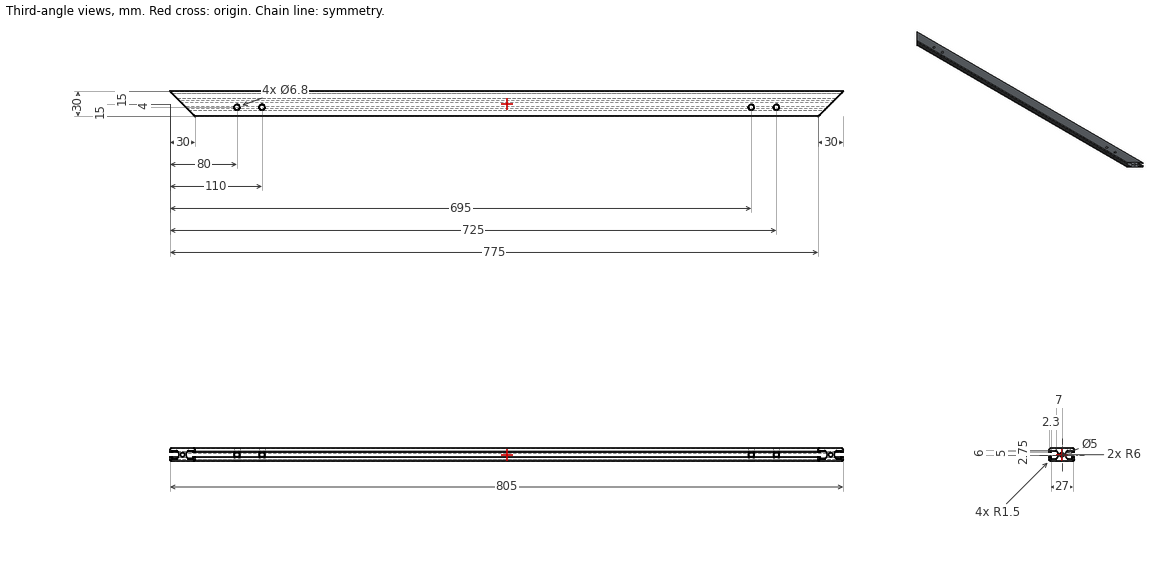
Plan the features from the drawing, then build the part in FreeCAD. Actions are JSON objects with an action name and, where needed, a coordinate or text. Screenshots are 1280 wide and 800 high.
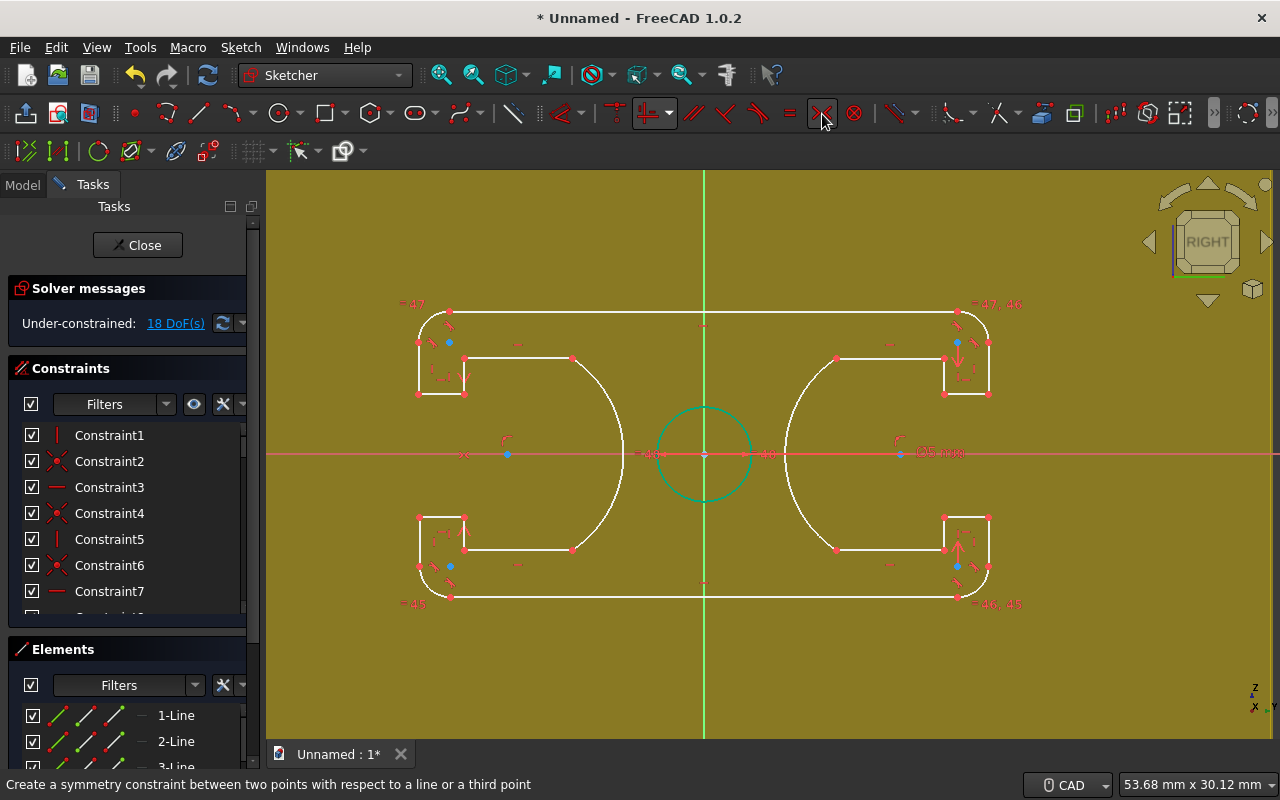
{"action": "left_click", "coordinate": [419, 394]}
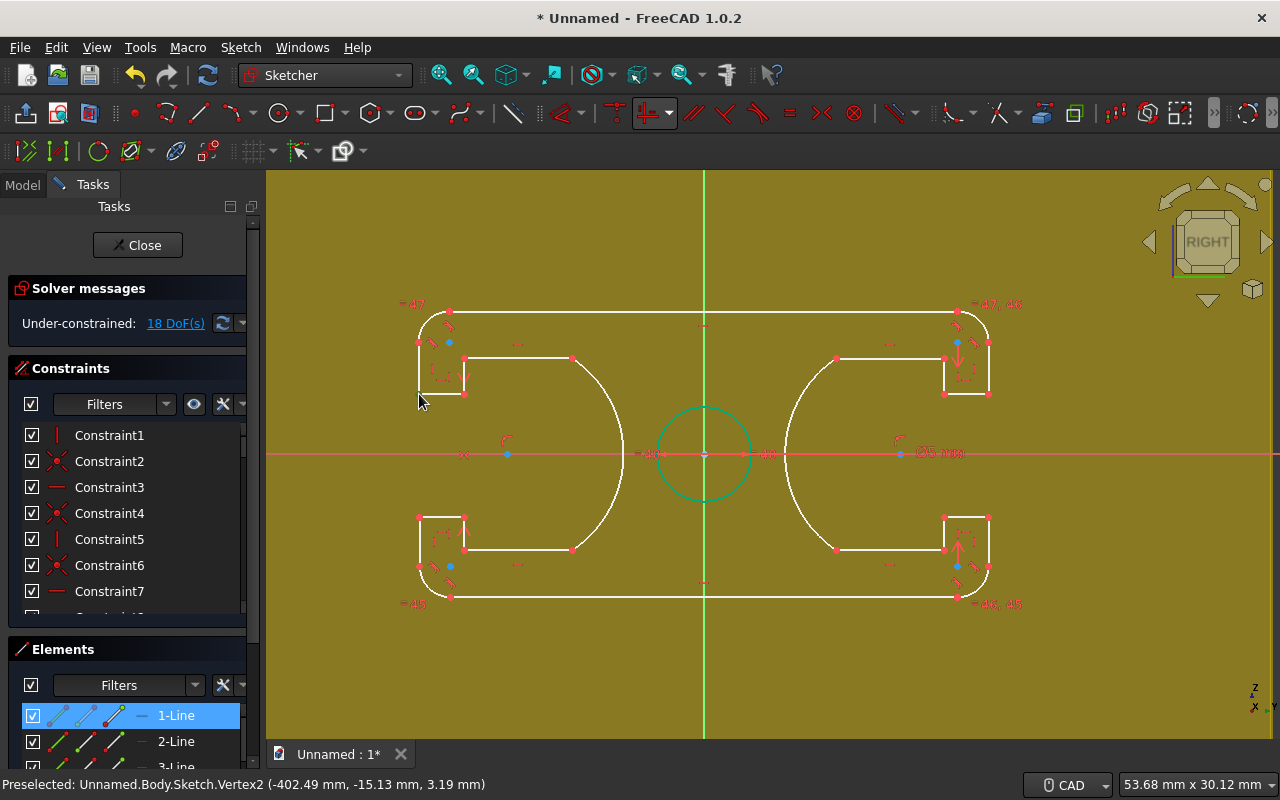
{"action": "left_click", "coordinate": [420, 517]}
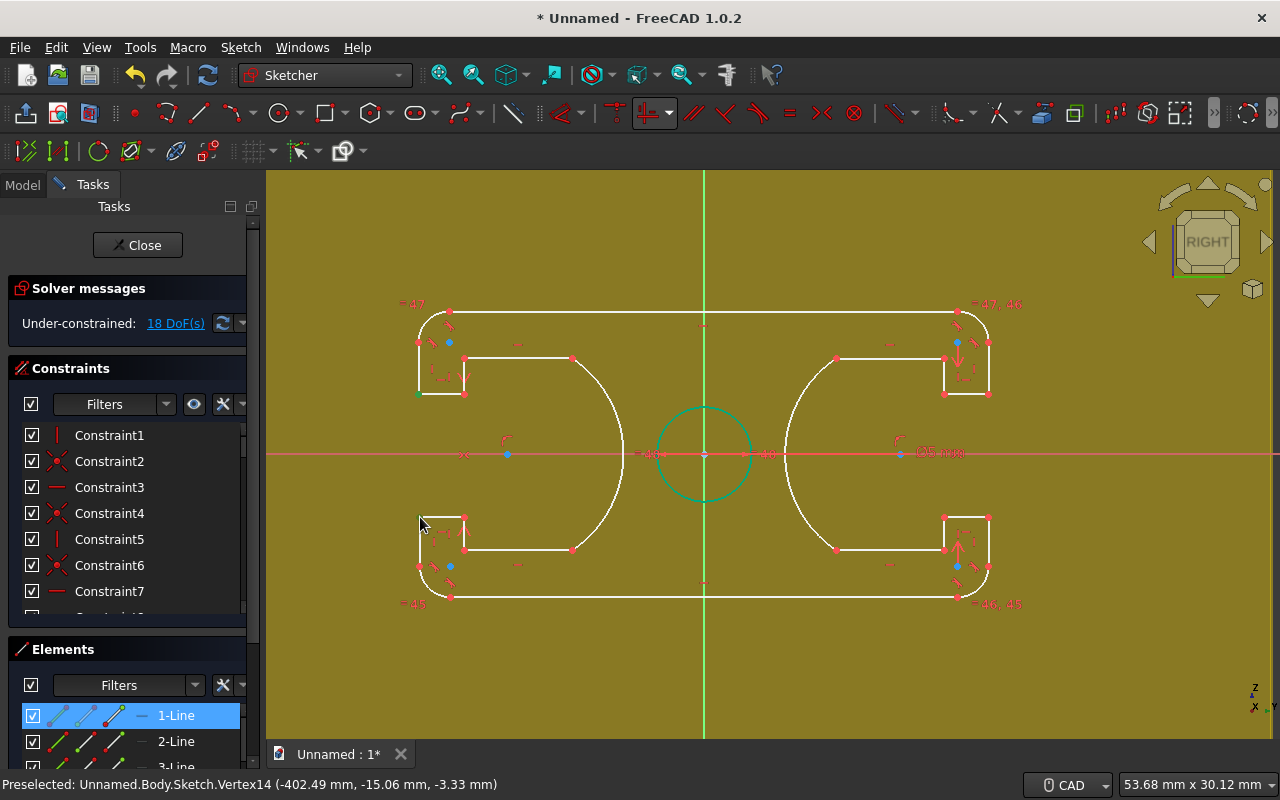
{"action": "left_click", "coordinate": [353, 454]}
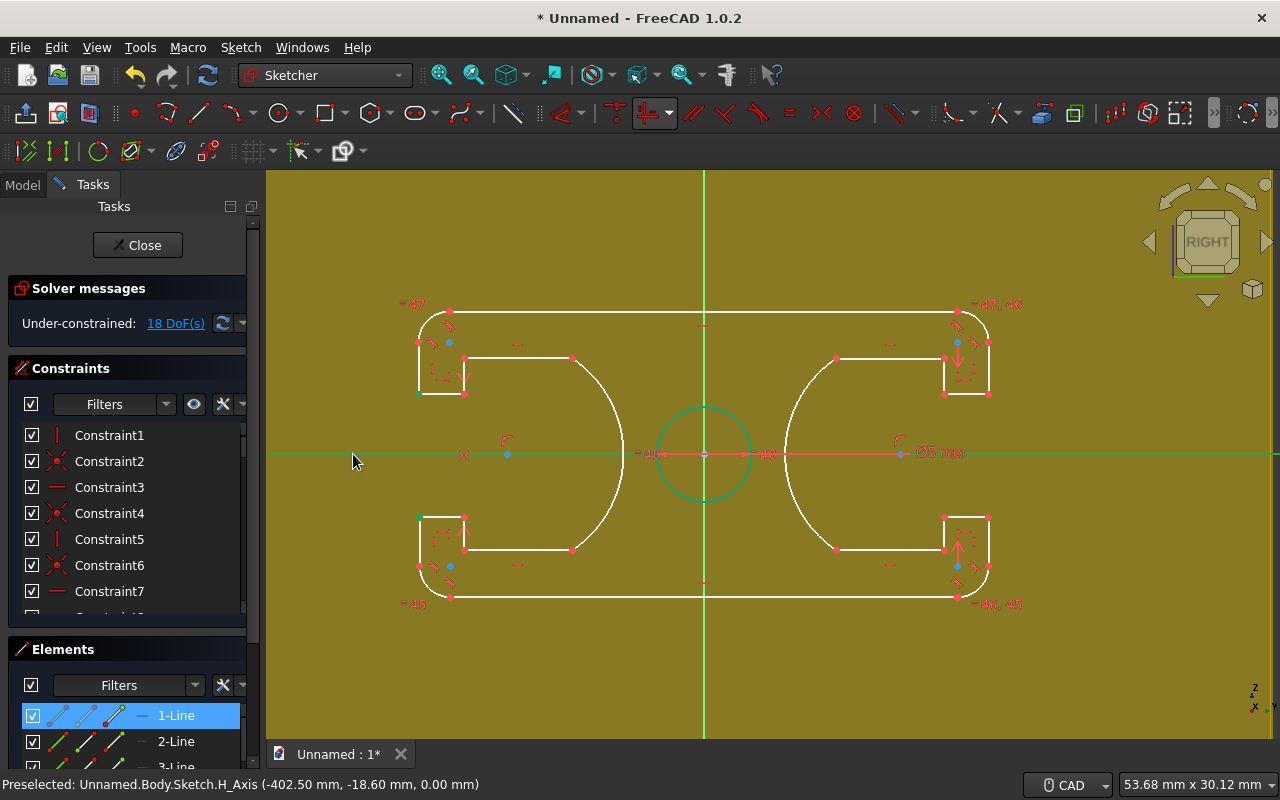
{"action": "left_click", "coordinate": [822, 114]}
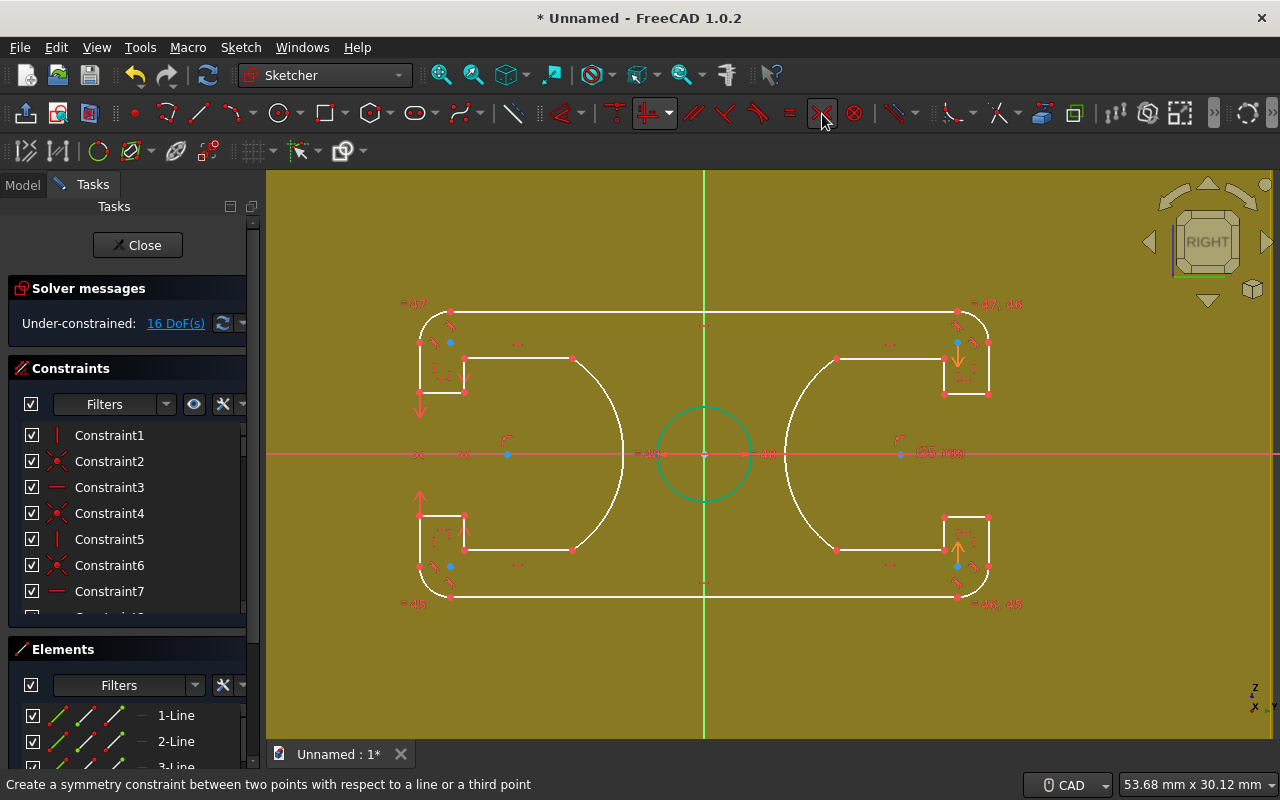
{"action": "left_click", "coordinate": [420, 516]}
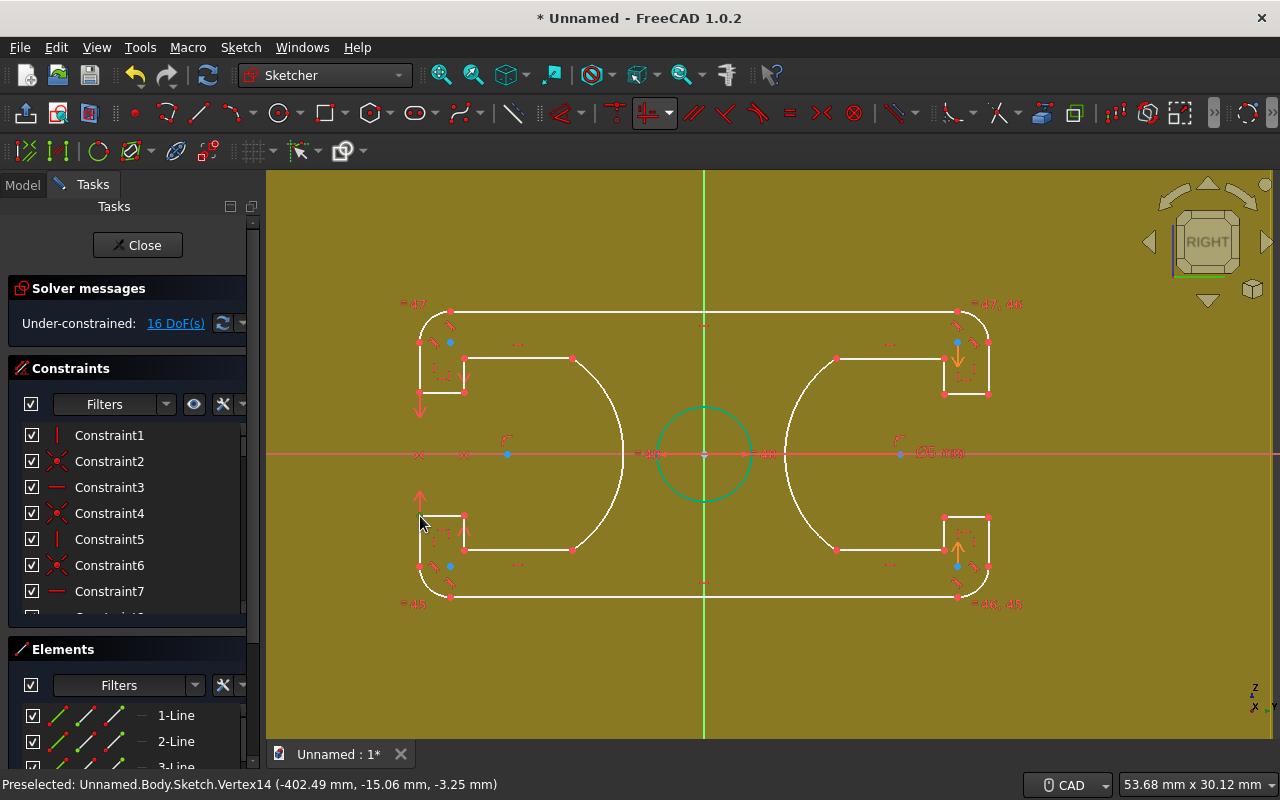
{"action": "left_click", "coordinate": [989, 517]}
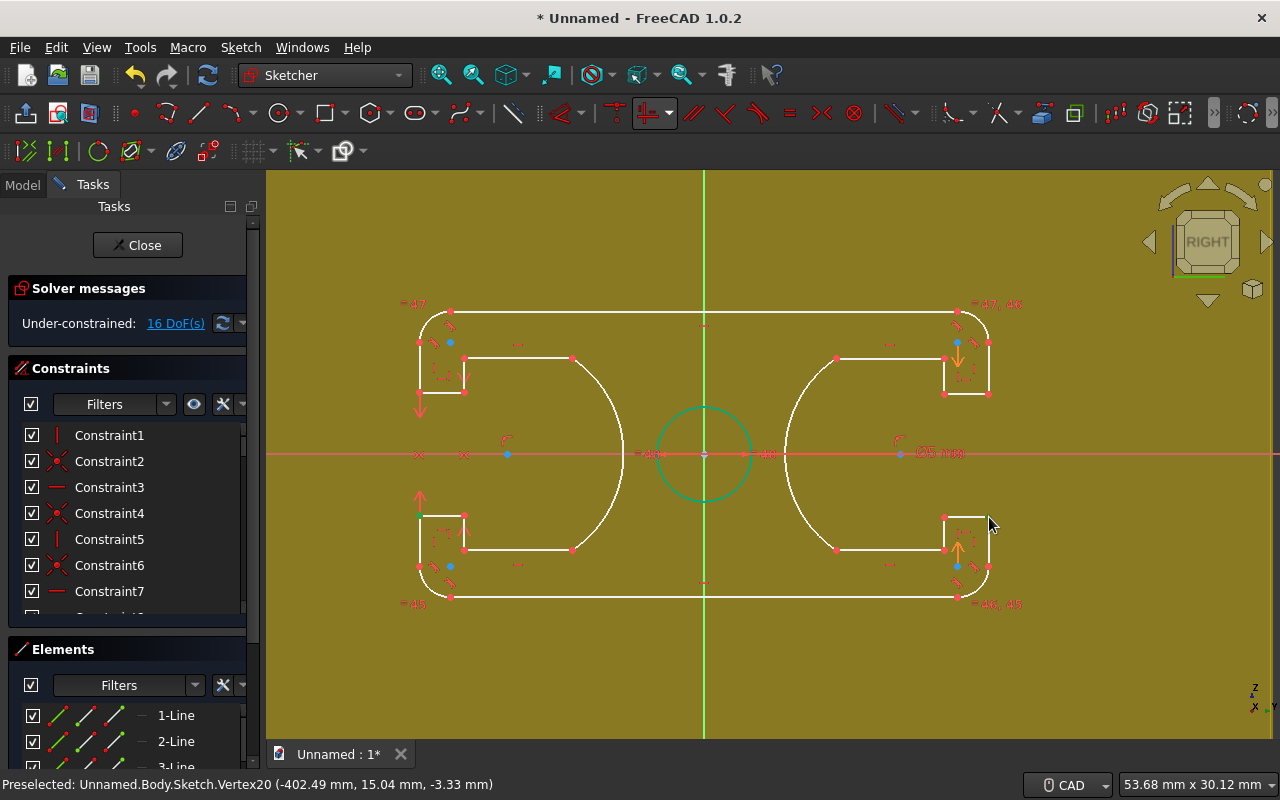
{"action": "left_click", "coordinate": [704, 674]}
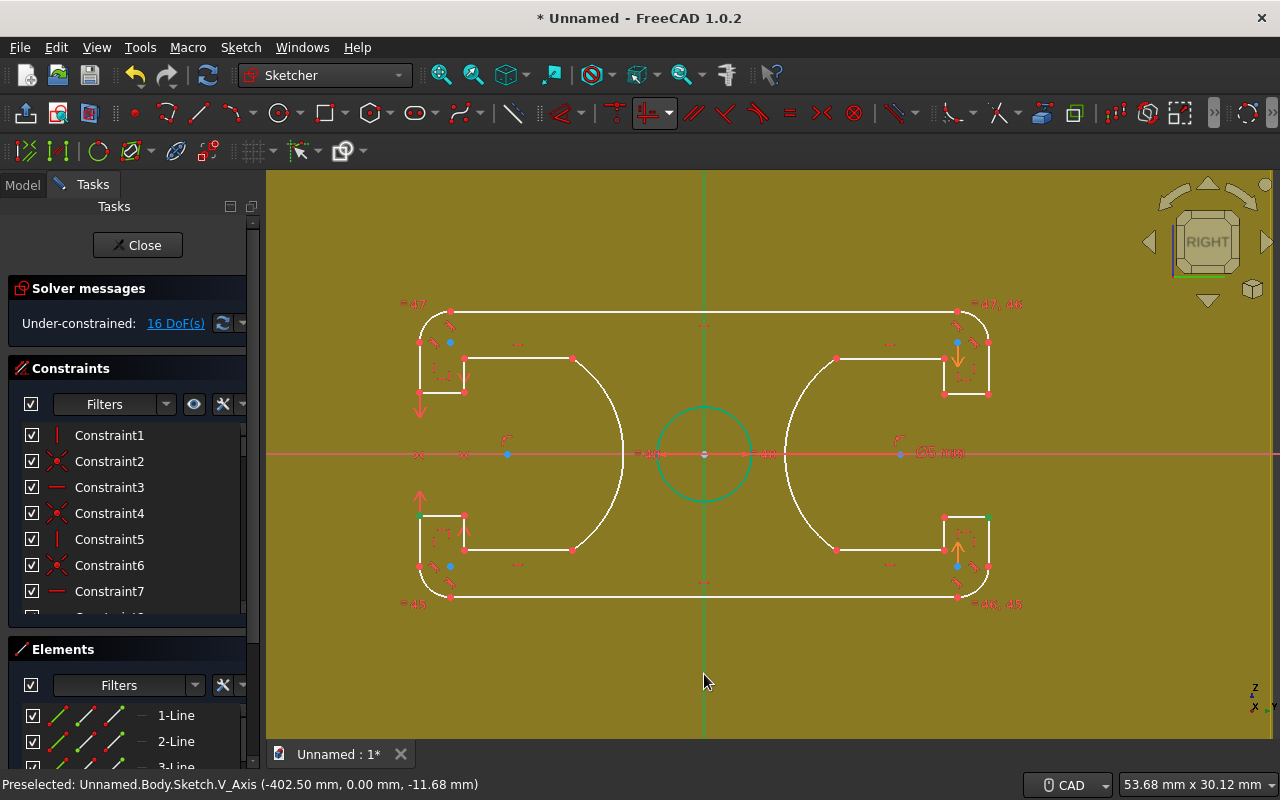
{"action": "left_click", "coordinate": [822, 114]}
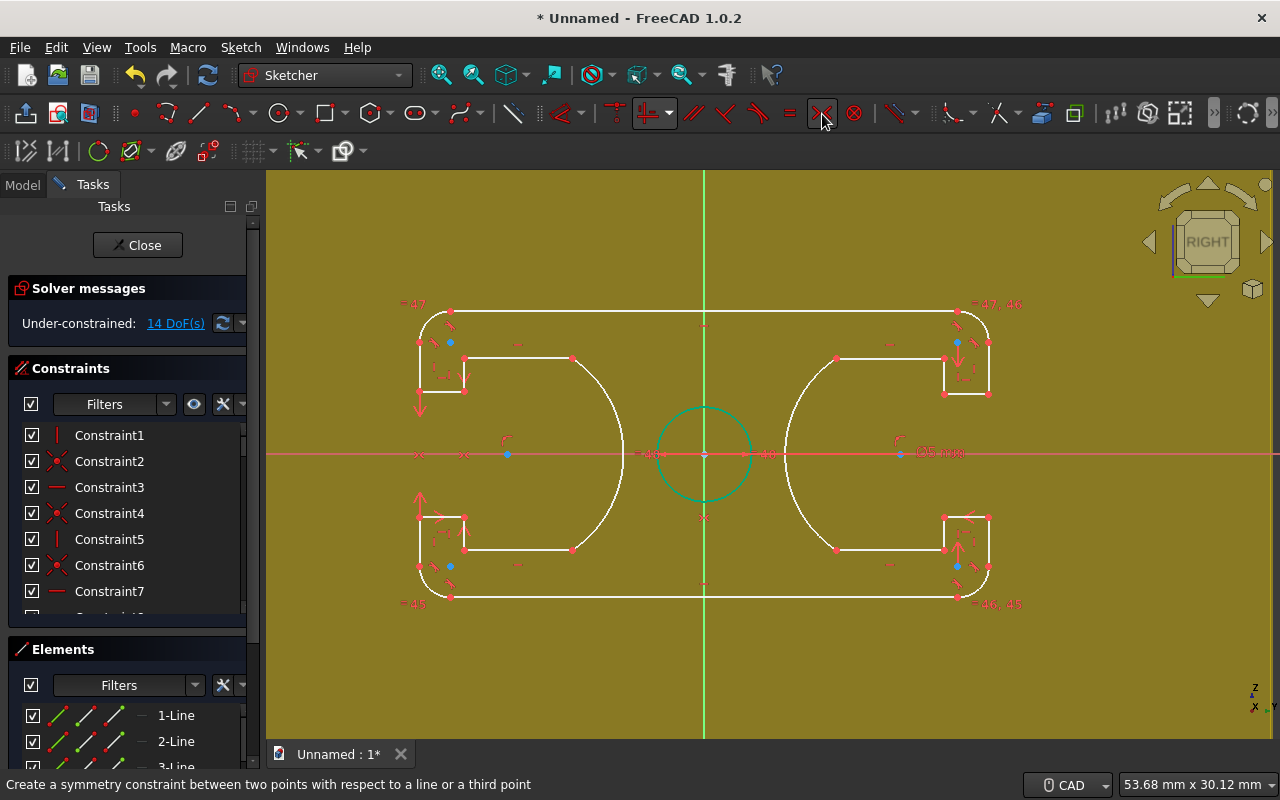
{"action": "left_click", "coordinate": [464, 550]}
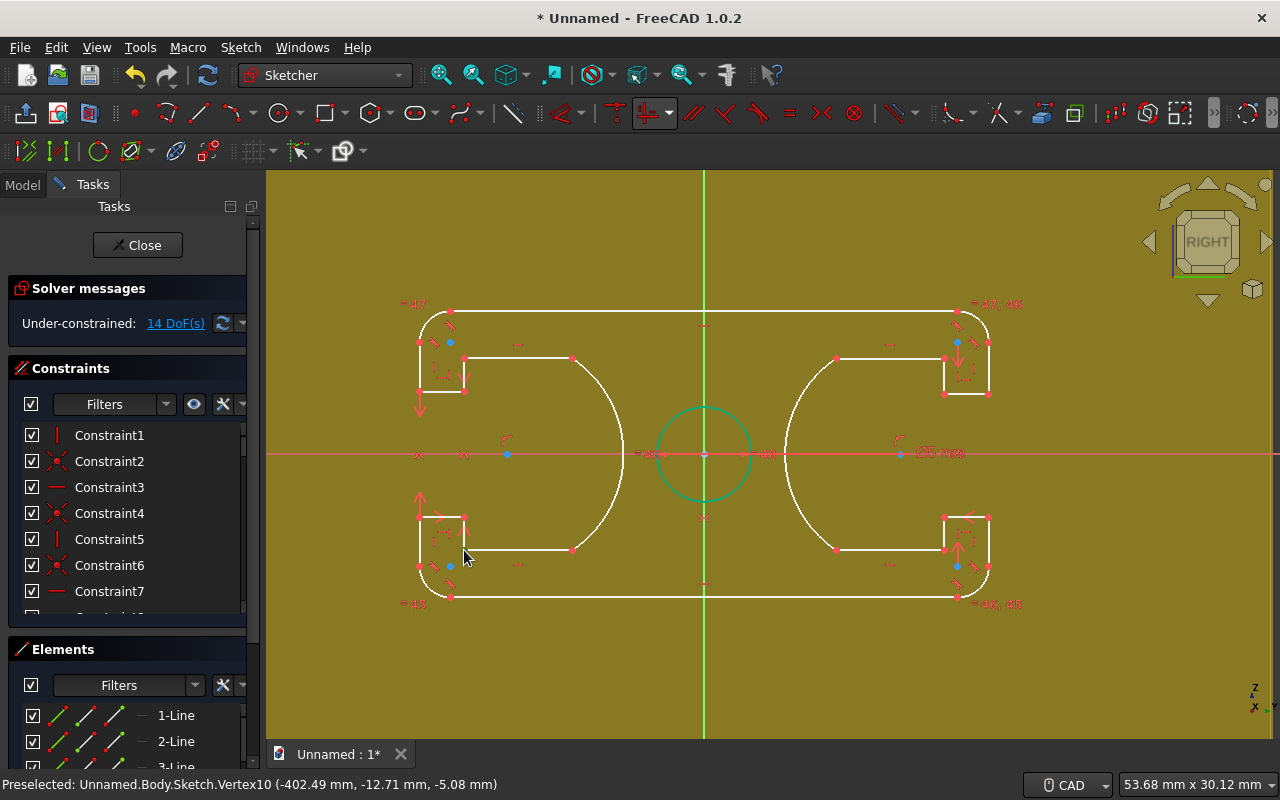
{"action": "left_click", "coordinate": [944, 550]}